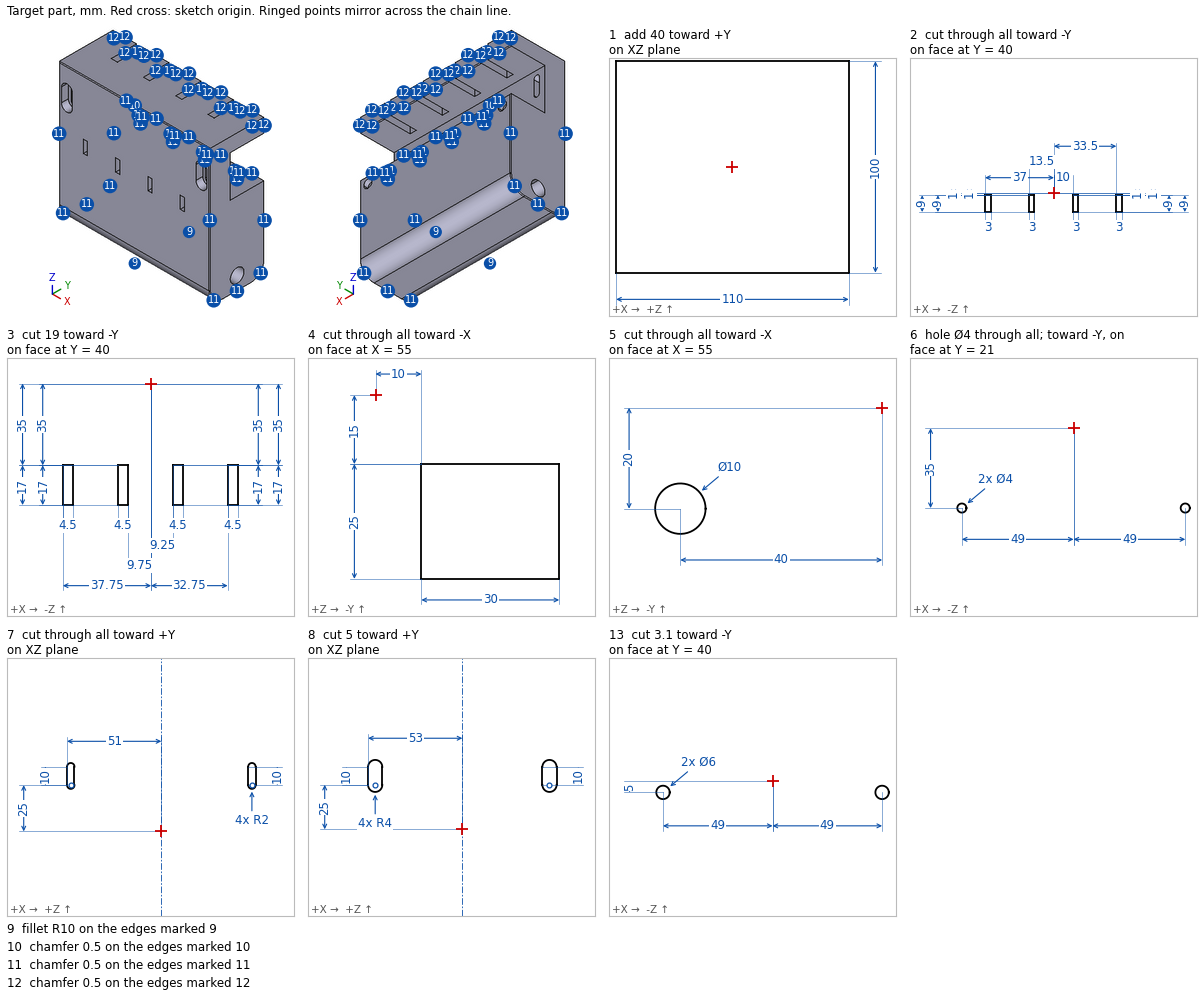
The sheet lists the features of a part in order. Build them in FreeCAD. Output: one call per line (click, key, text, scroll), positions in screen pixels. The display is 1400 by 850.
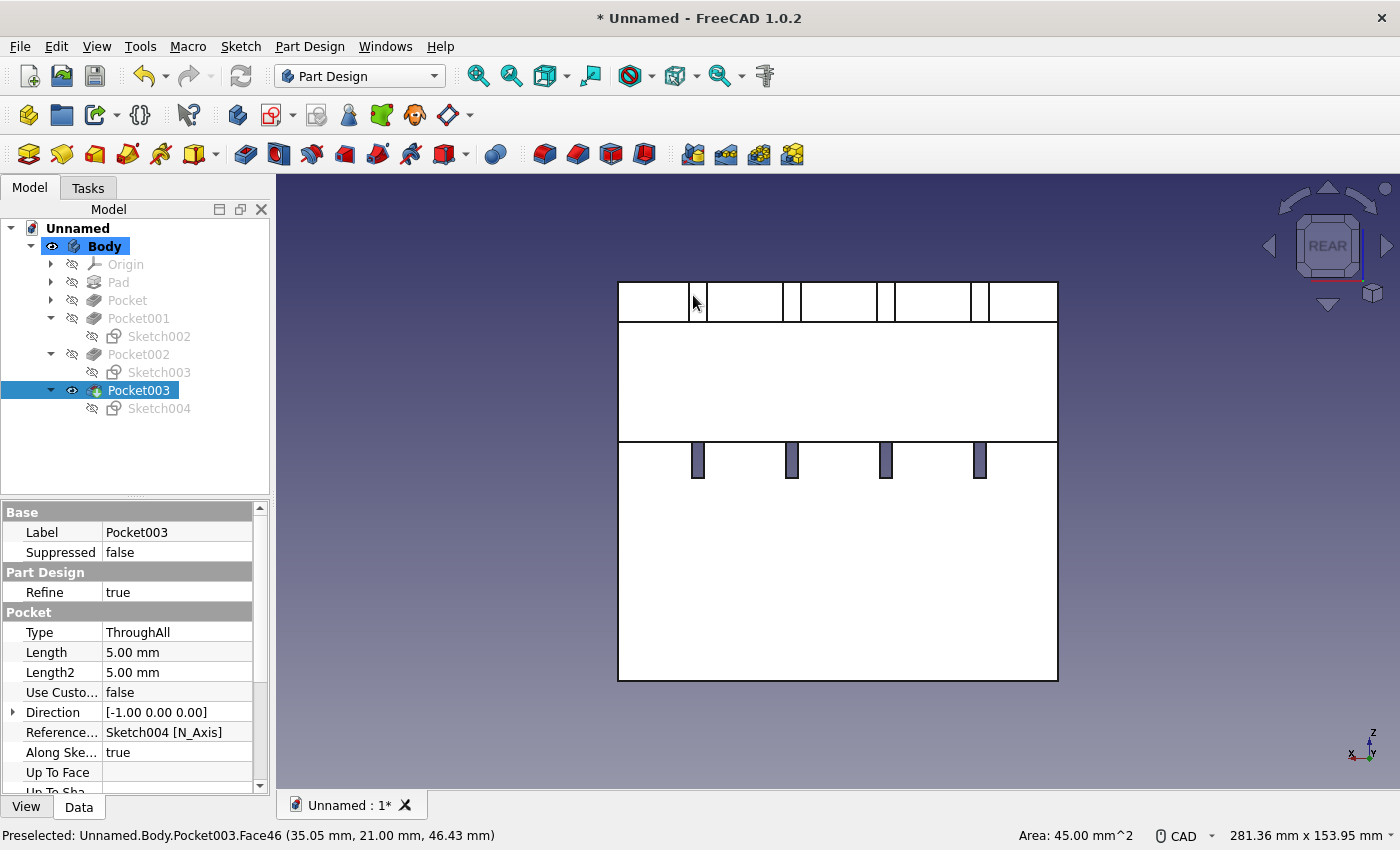
click(270, 116)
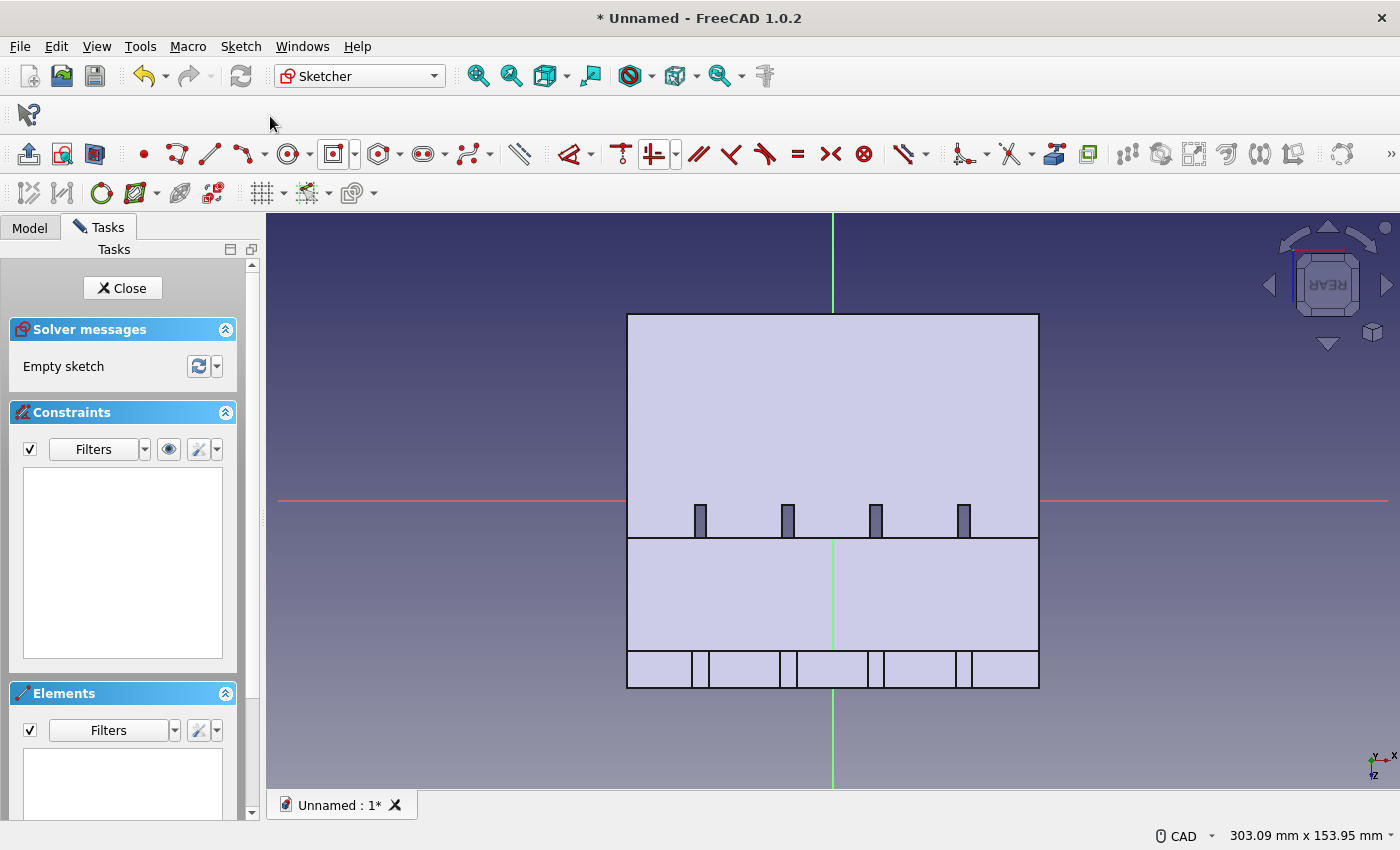
key(q)
key(s)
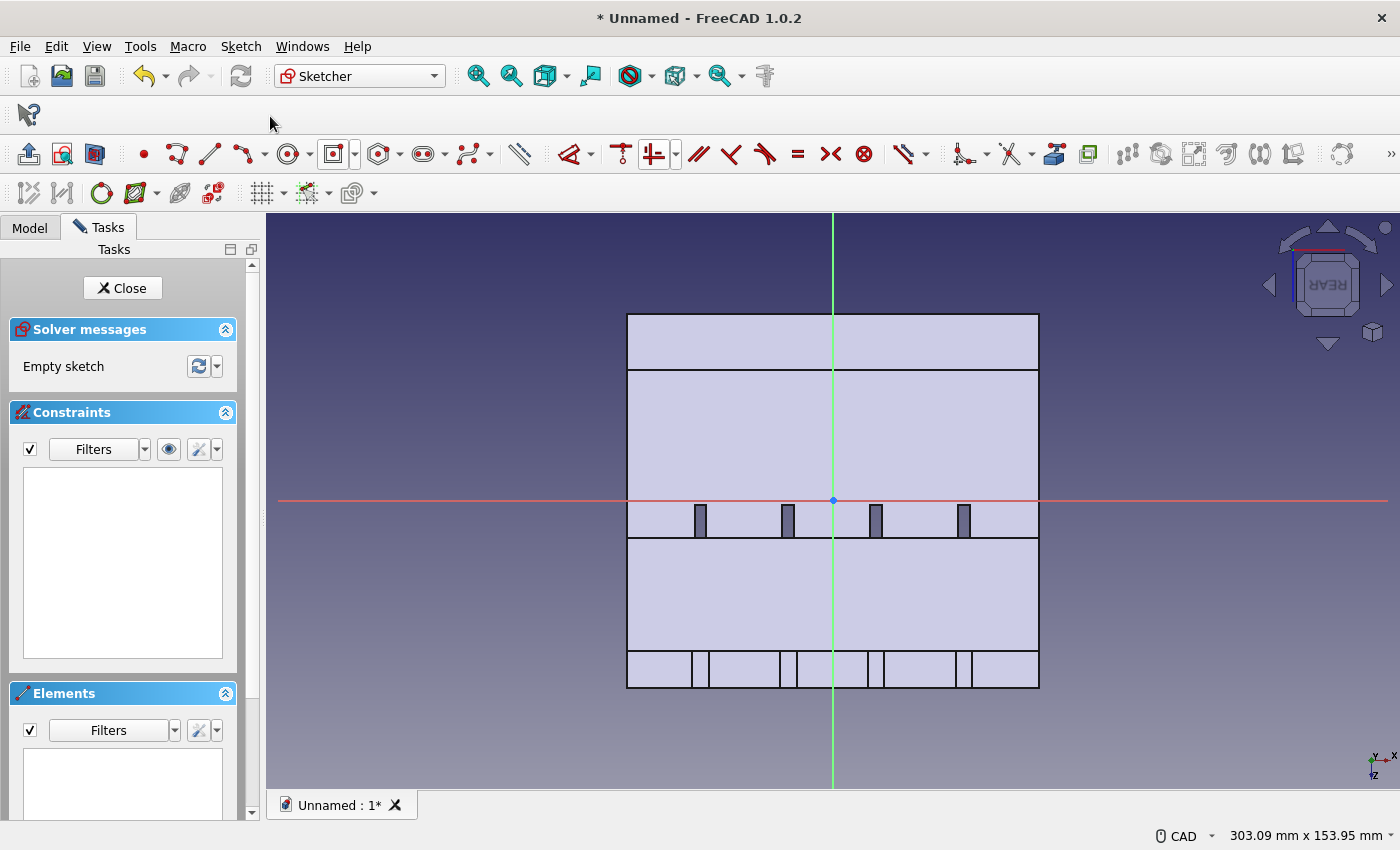
scroll(916, 654, up, 3)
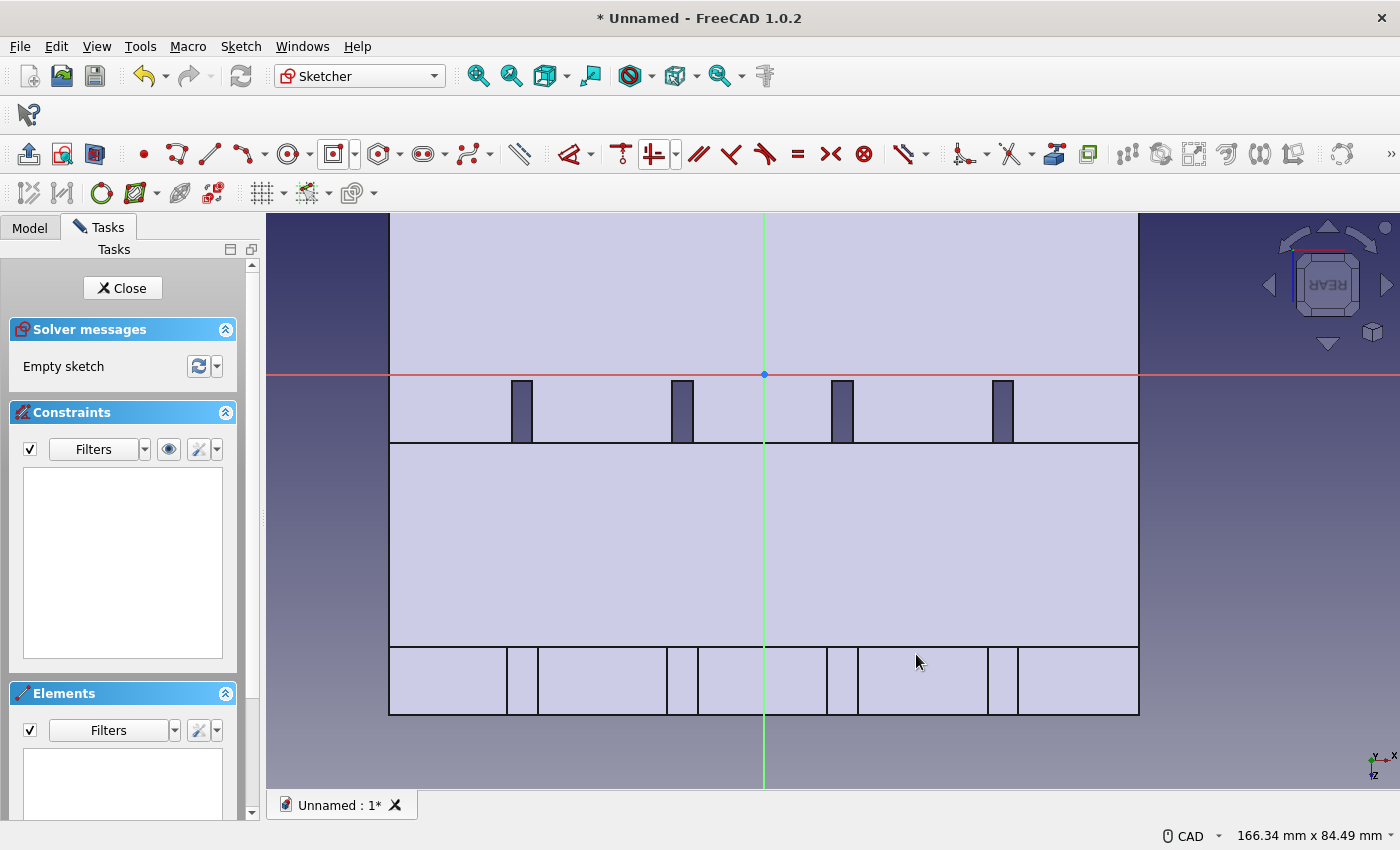
key(g)
key(c)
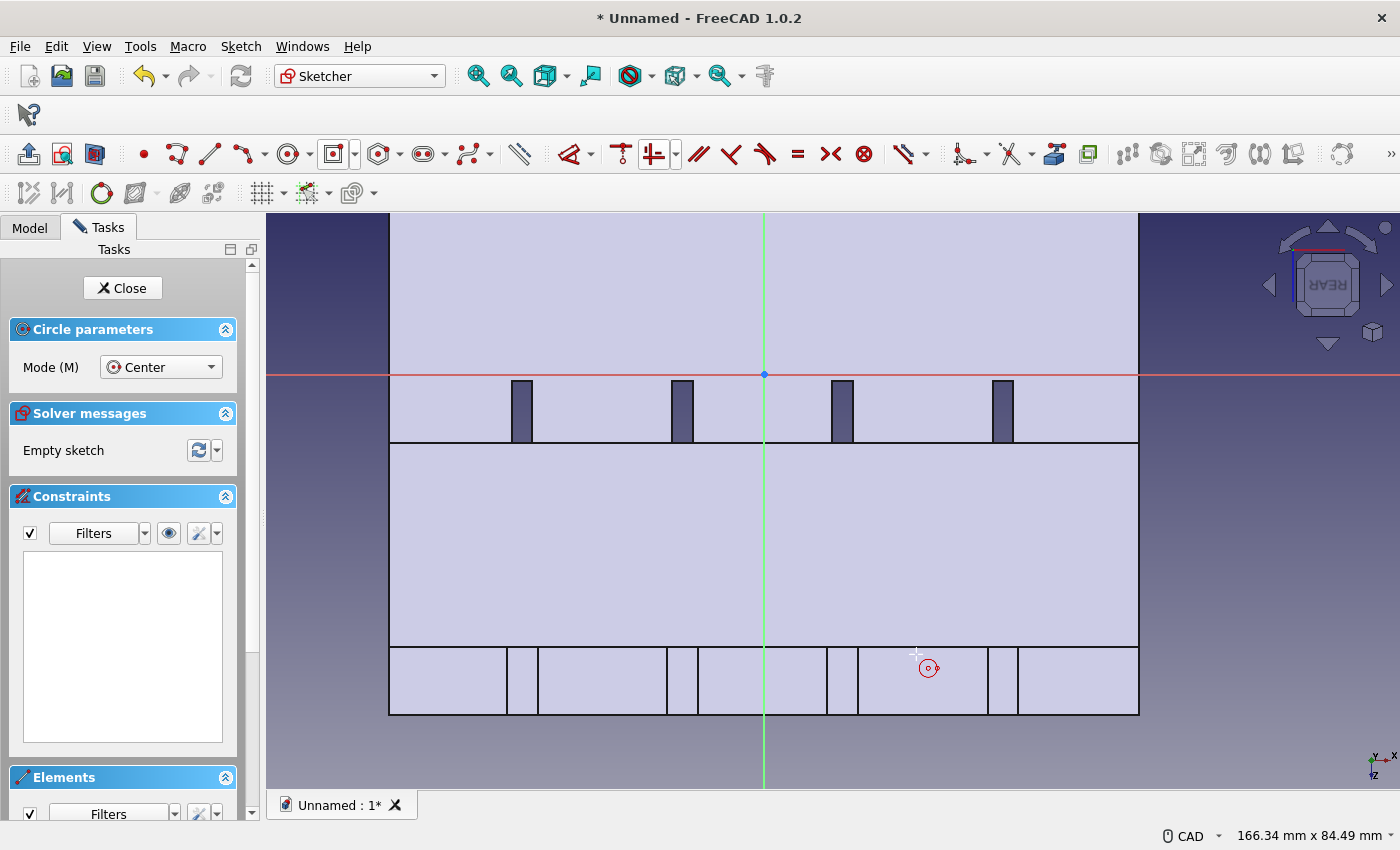
scroll(430, 613, up, 3)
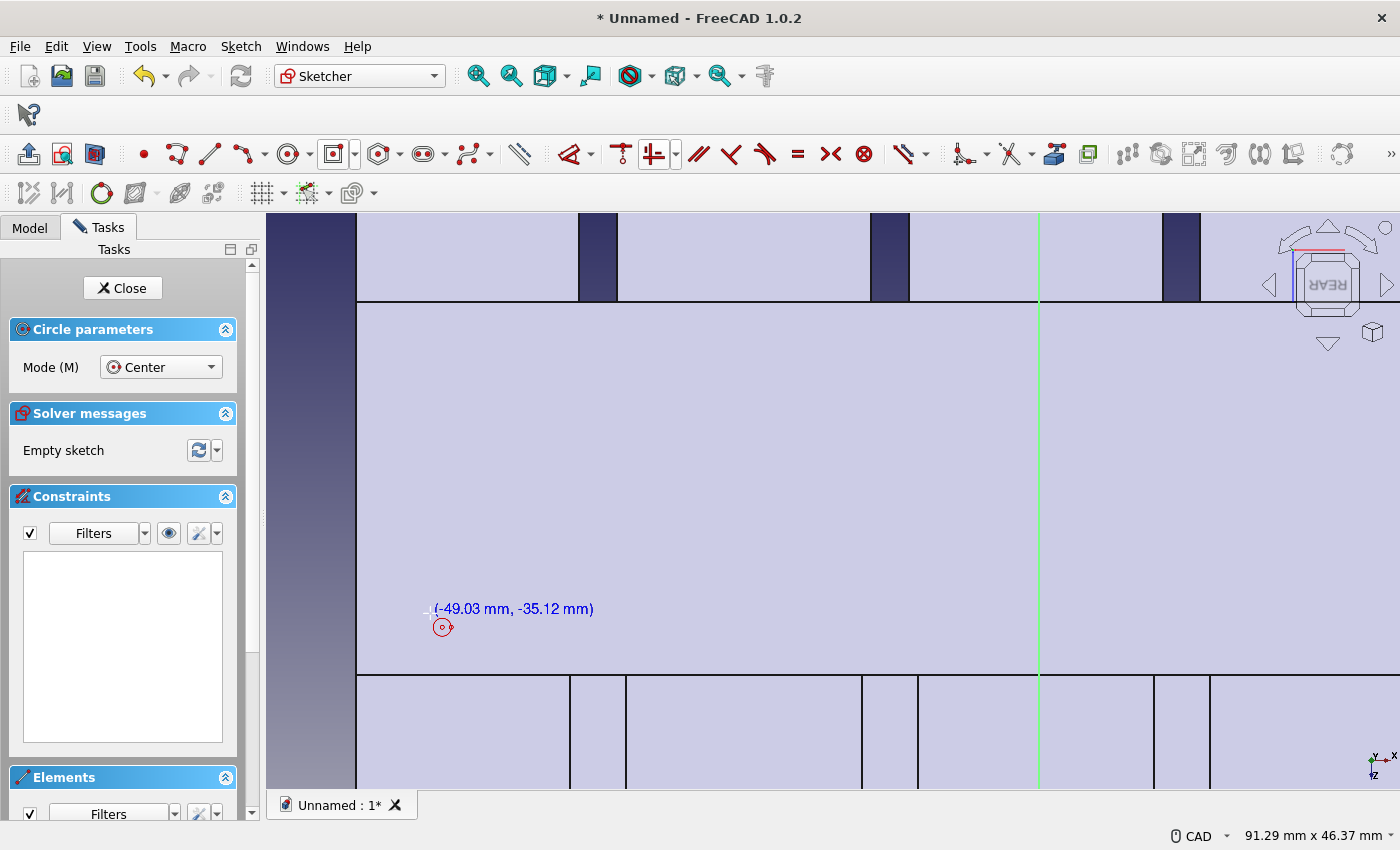
click(430, 613)
click(448, 595)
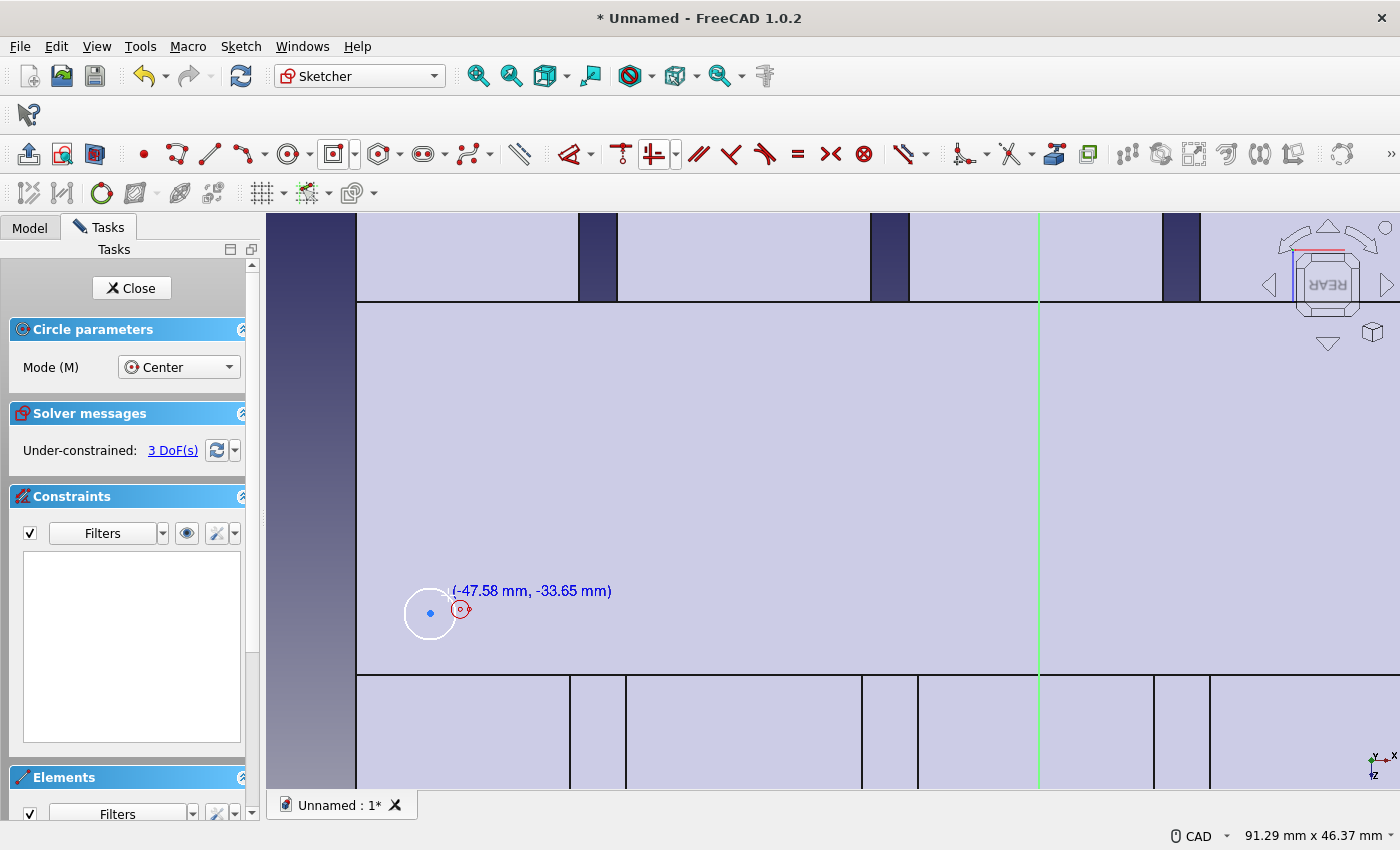
scroll(431, 614, down, 3)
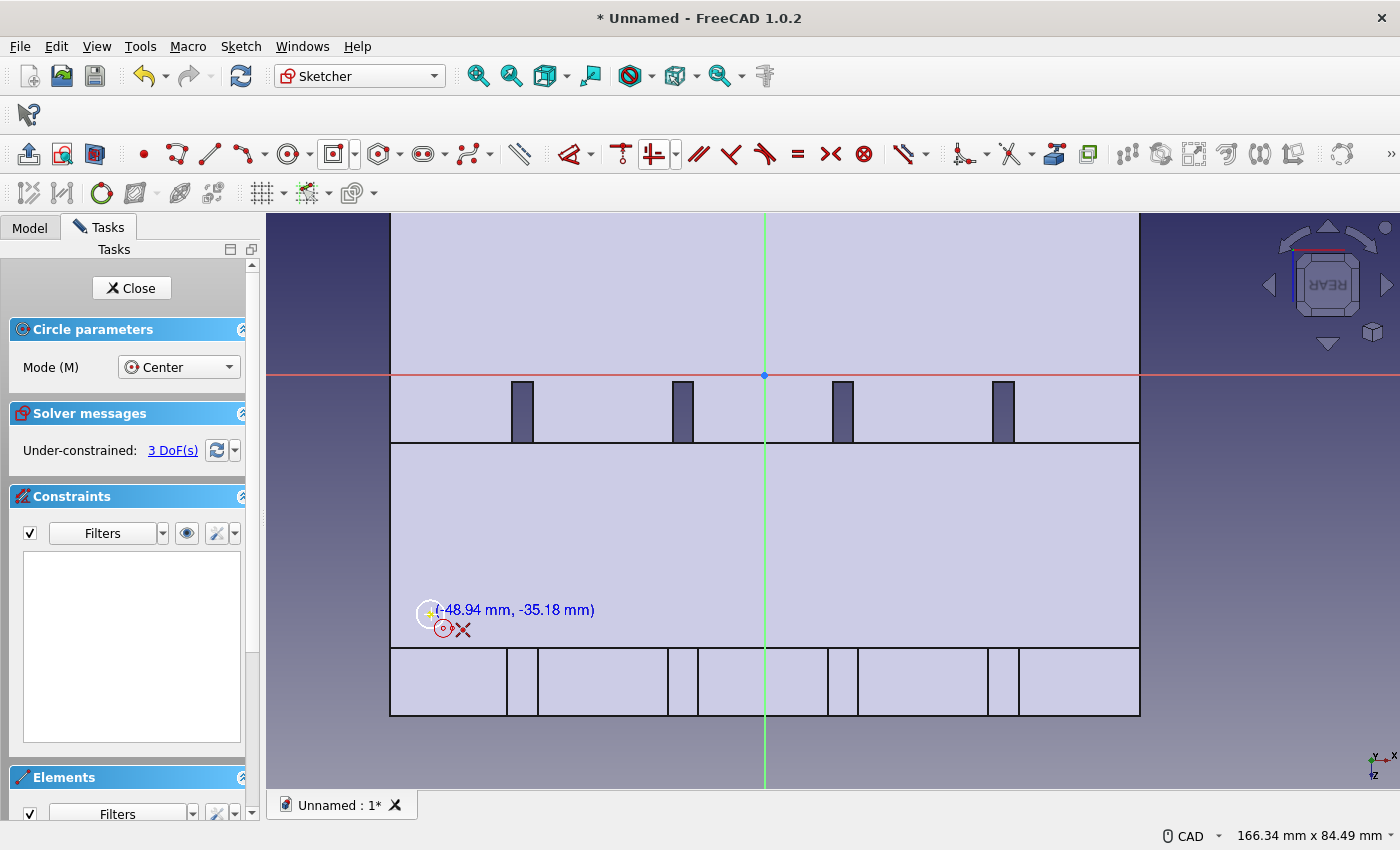
scroll(1099, 614, up, 3)